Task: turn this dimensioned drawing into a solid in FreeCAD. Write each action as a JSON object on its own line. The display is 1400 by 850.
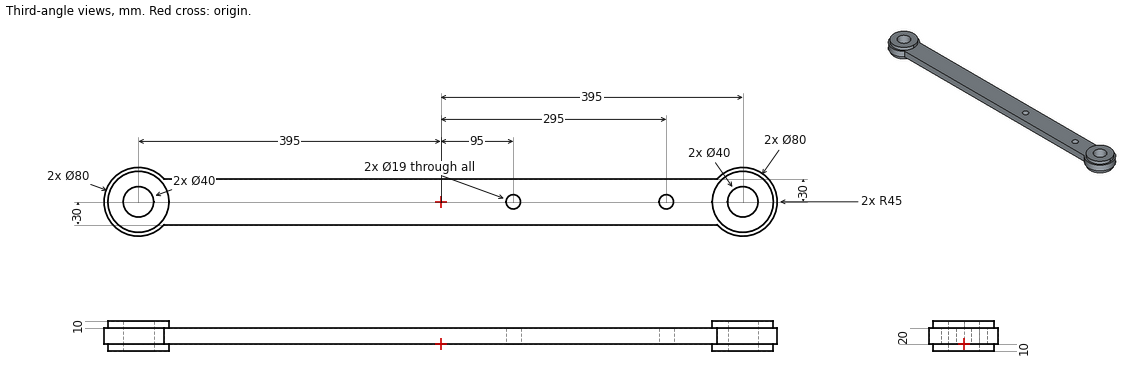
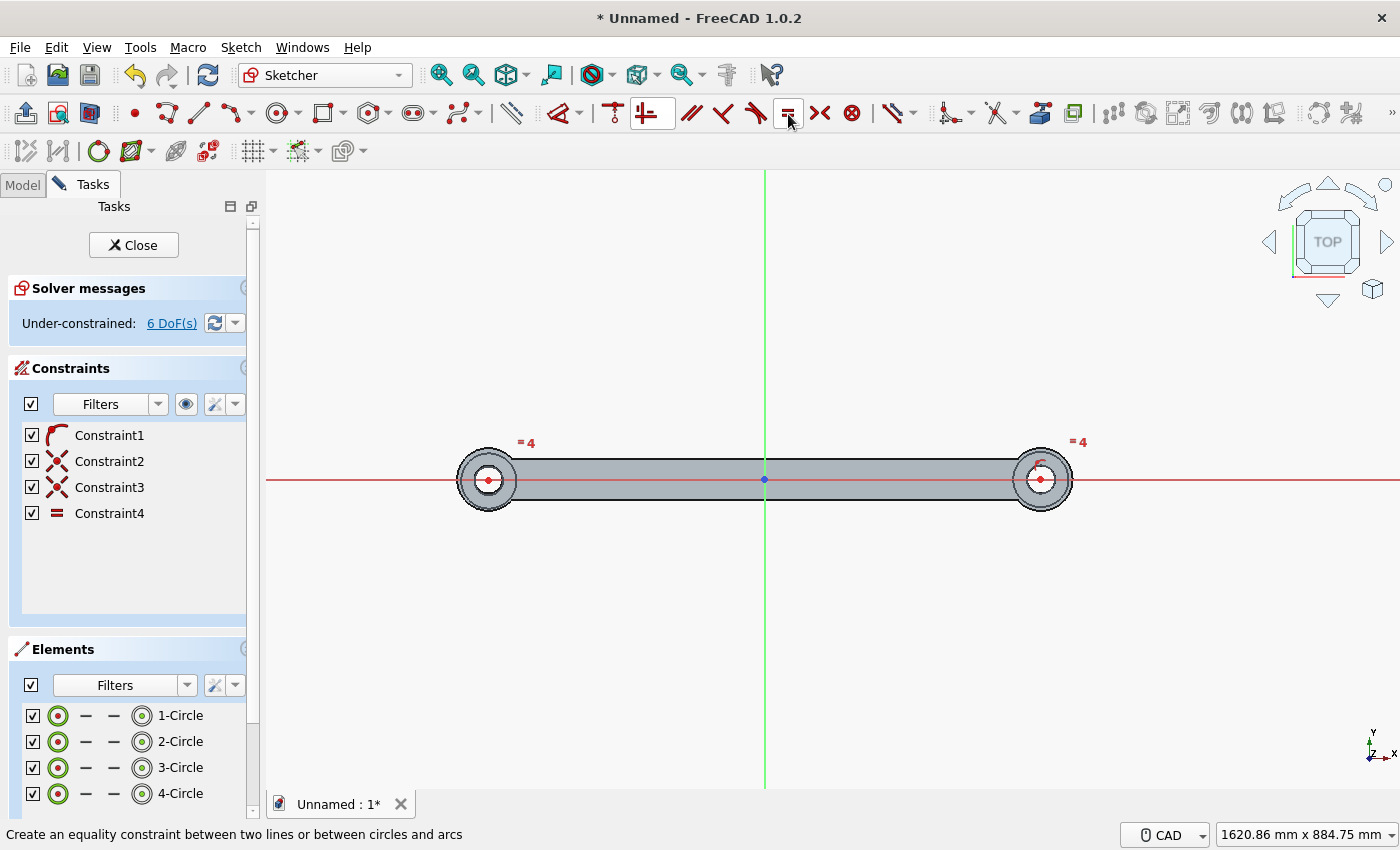
{"action": "left_click", "coordinate": [479, 491]}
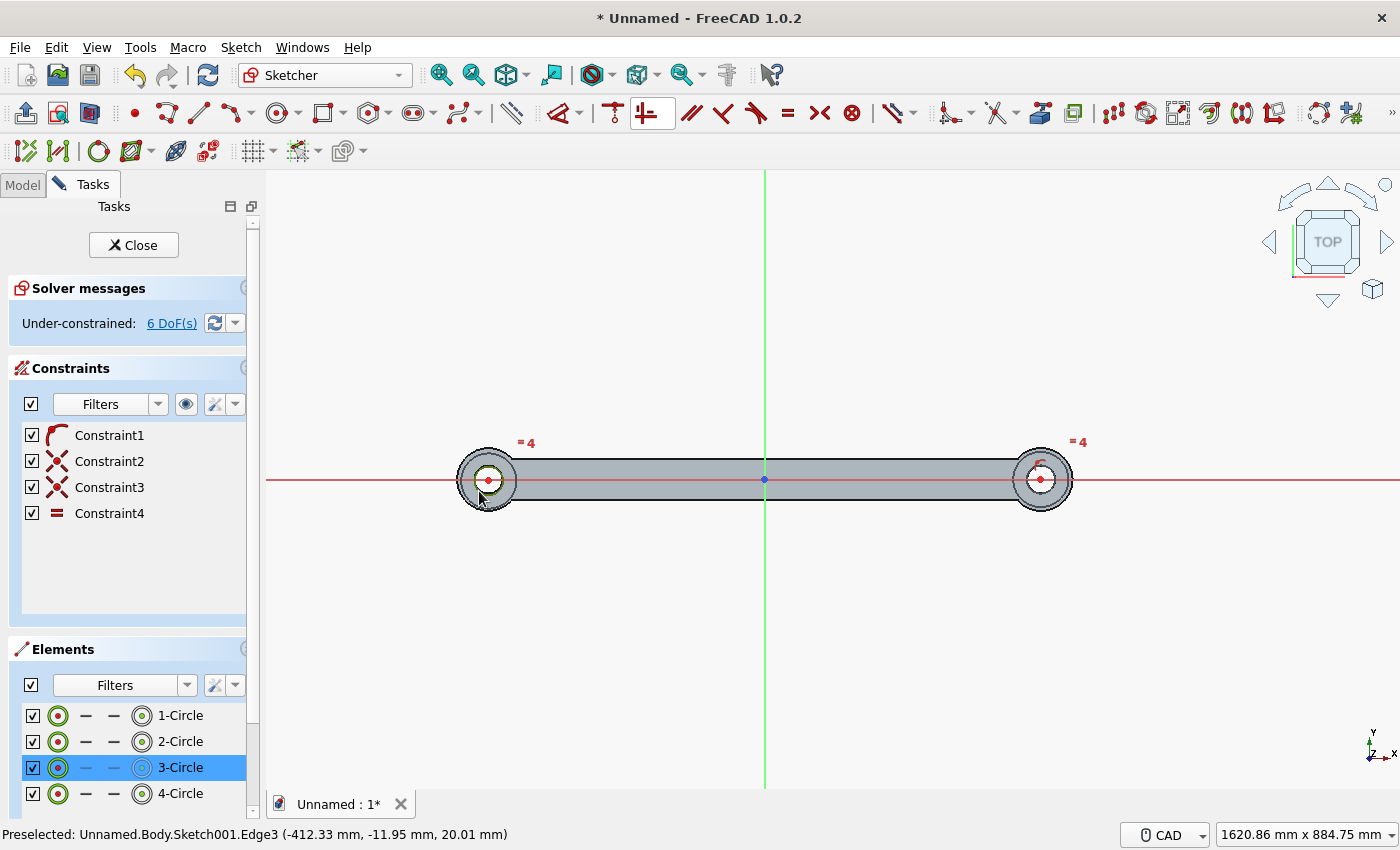
{"action": "scroll", "coordinate": [1051, 470], "scroll_direction": "up", "scroll_amount": 2}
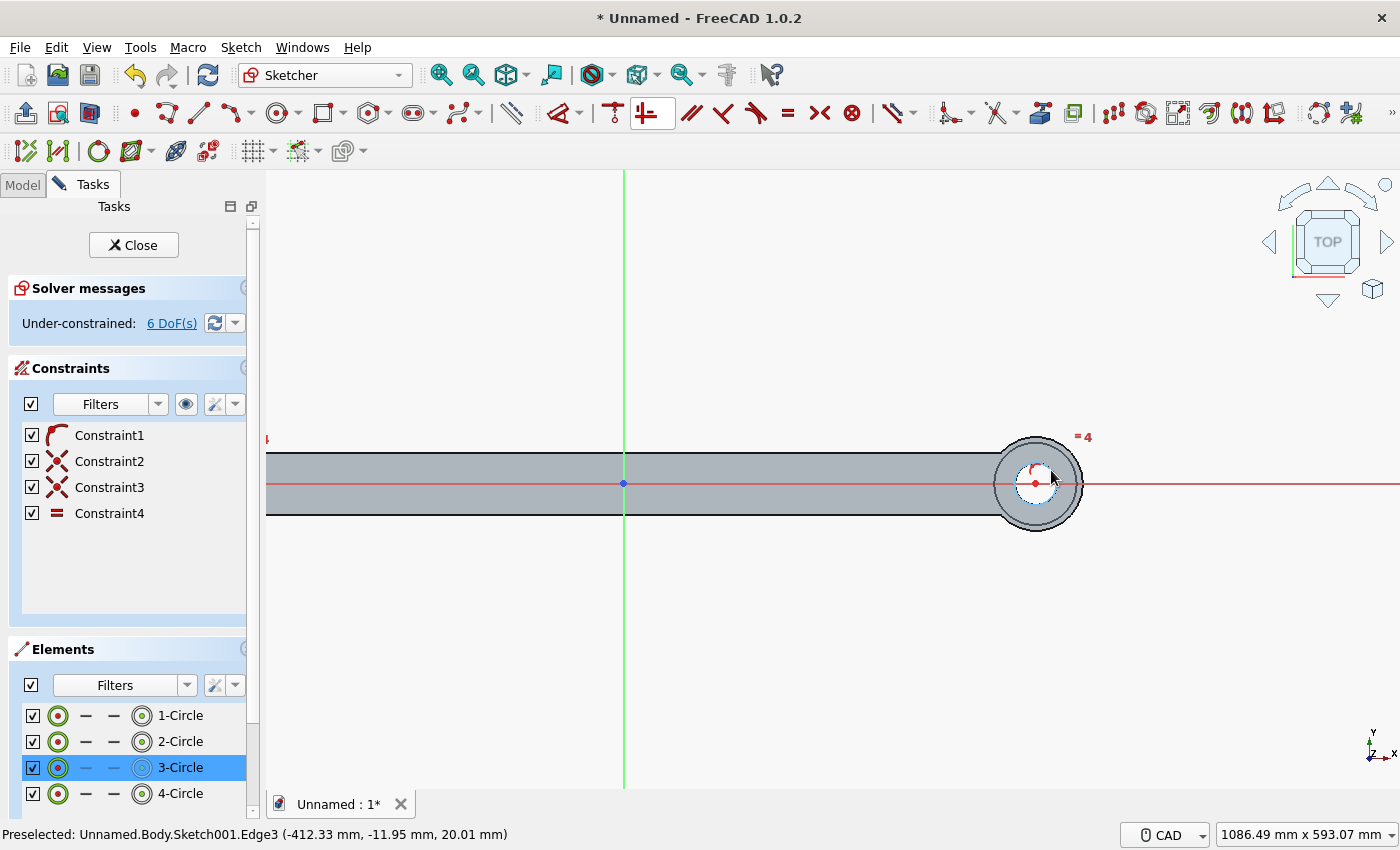
{"action": "left_click", "coordinate": [1050, 469]}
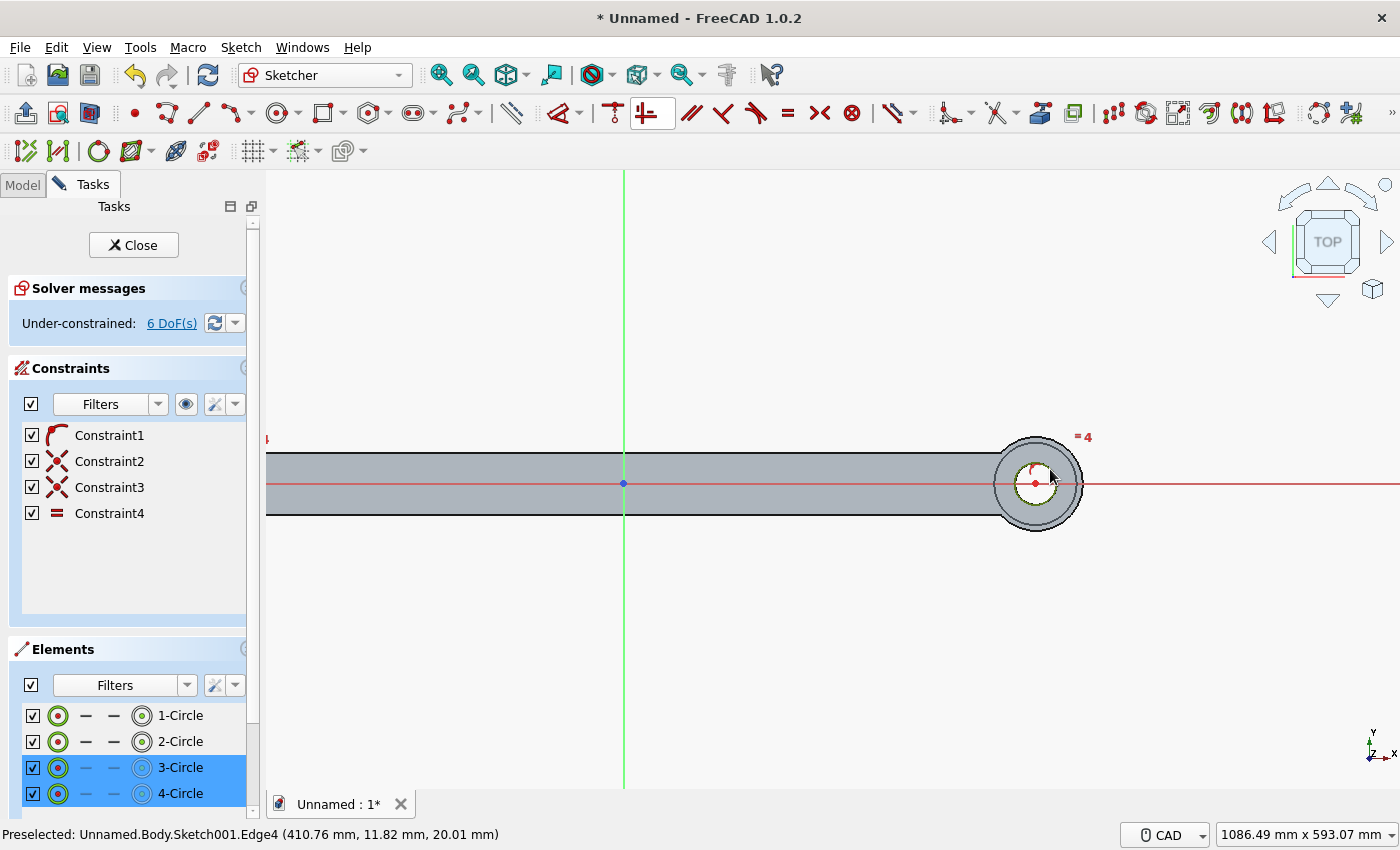
{"action": "left_click", "coordinate": [788, 114]}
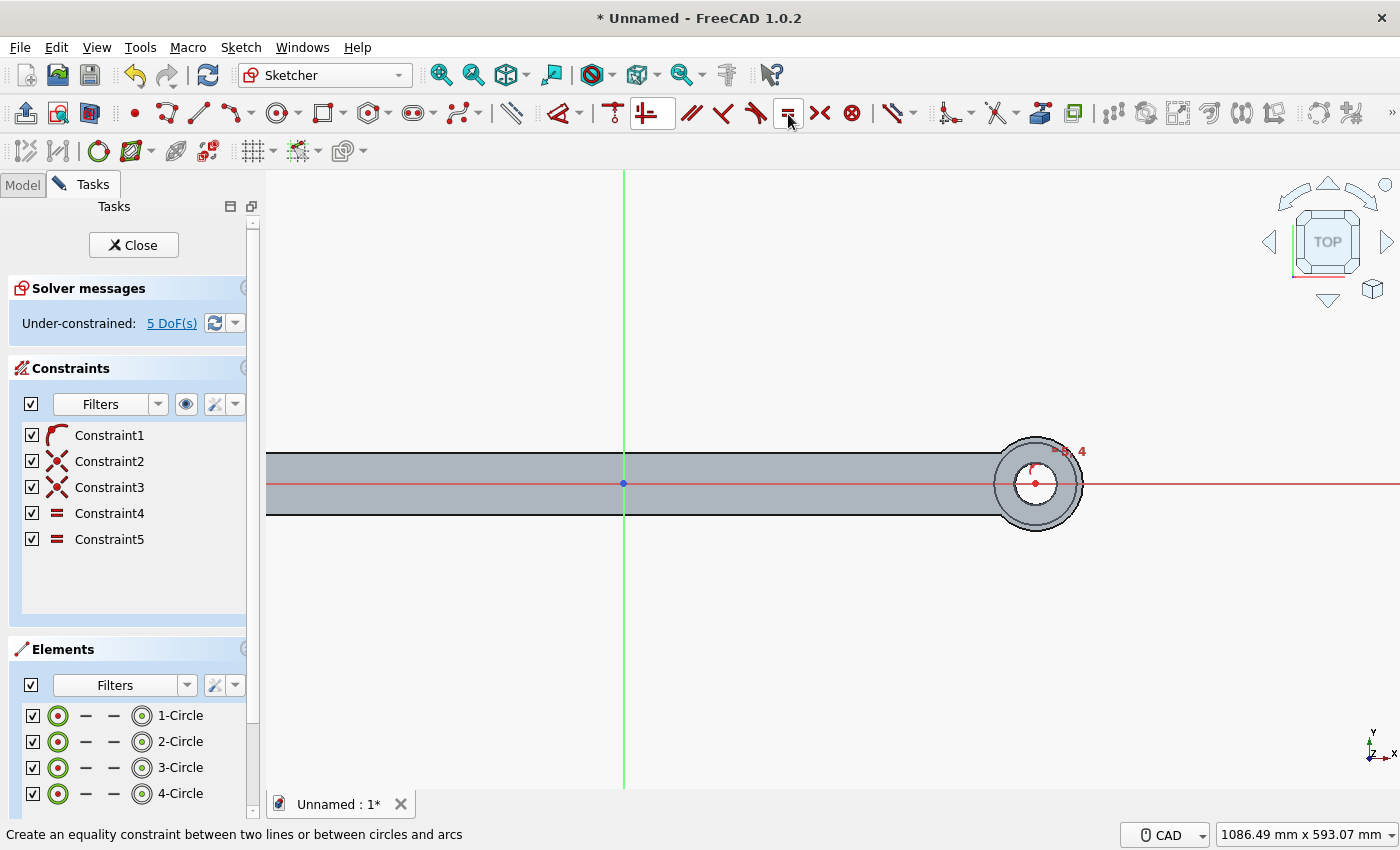
{"action": "scroll", "coordinate": [1051, 470], "scroll_direction": "down", "scroll_amount": 2}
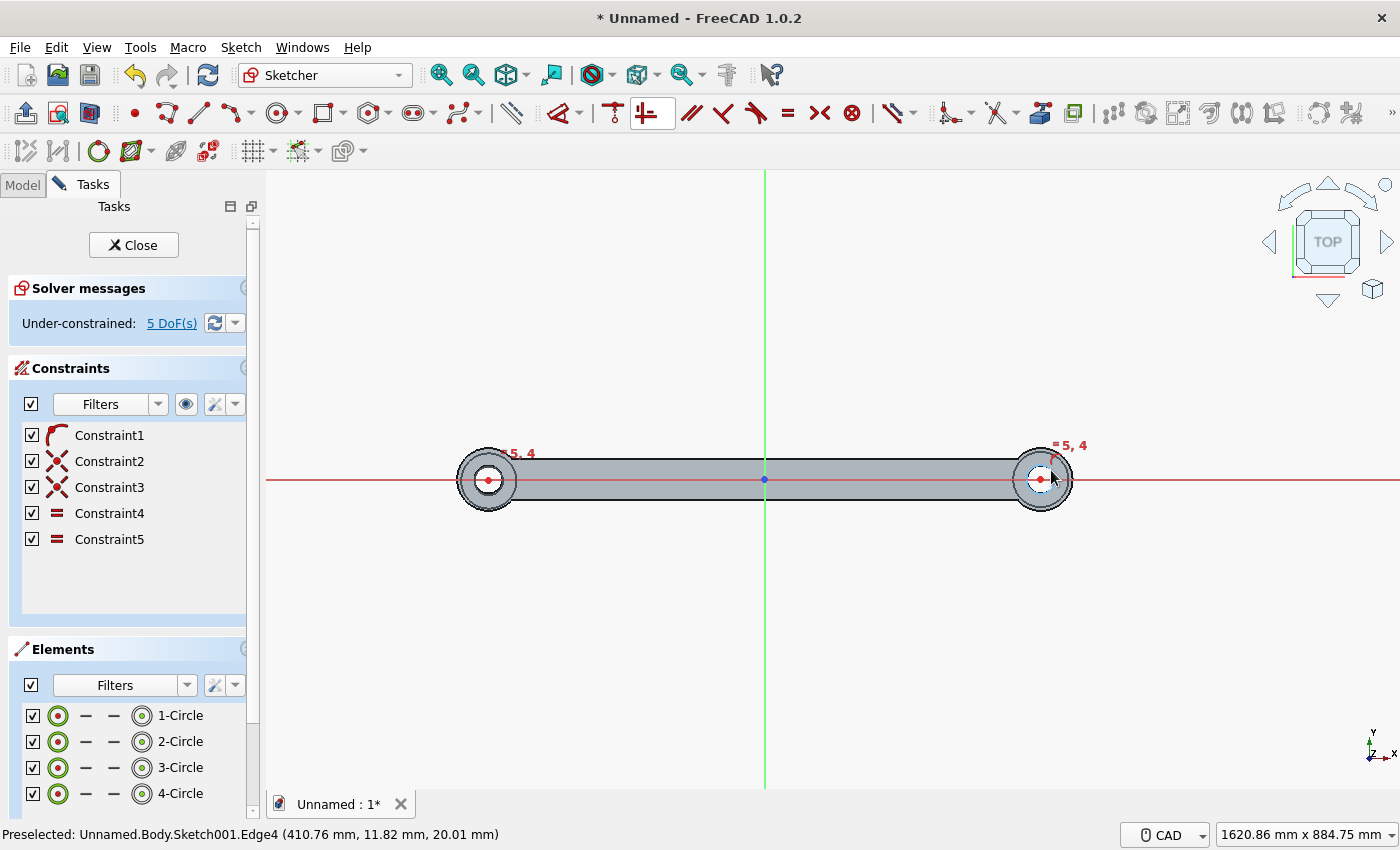
{"action": "left_click", "coordinate": [489, 481]}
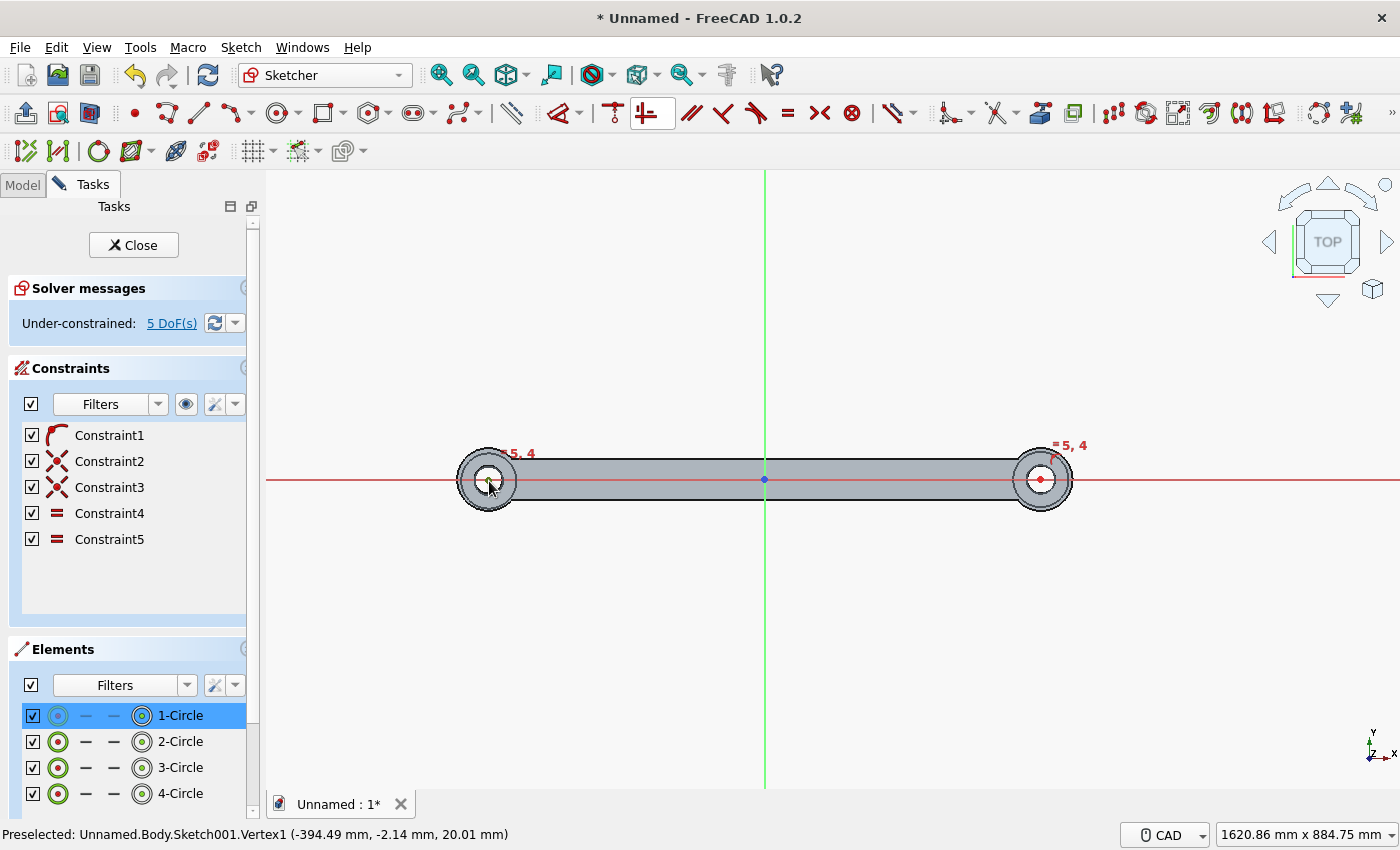
{"action": "left_click", "coordinate": [361, 480]}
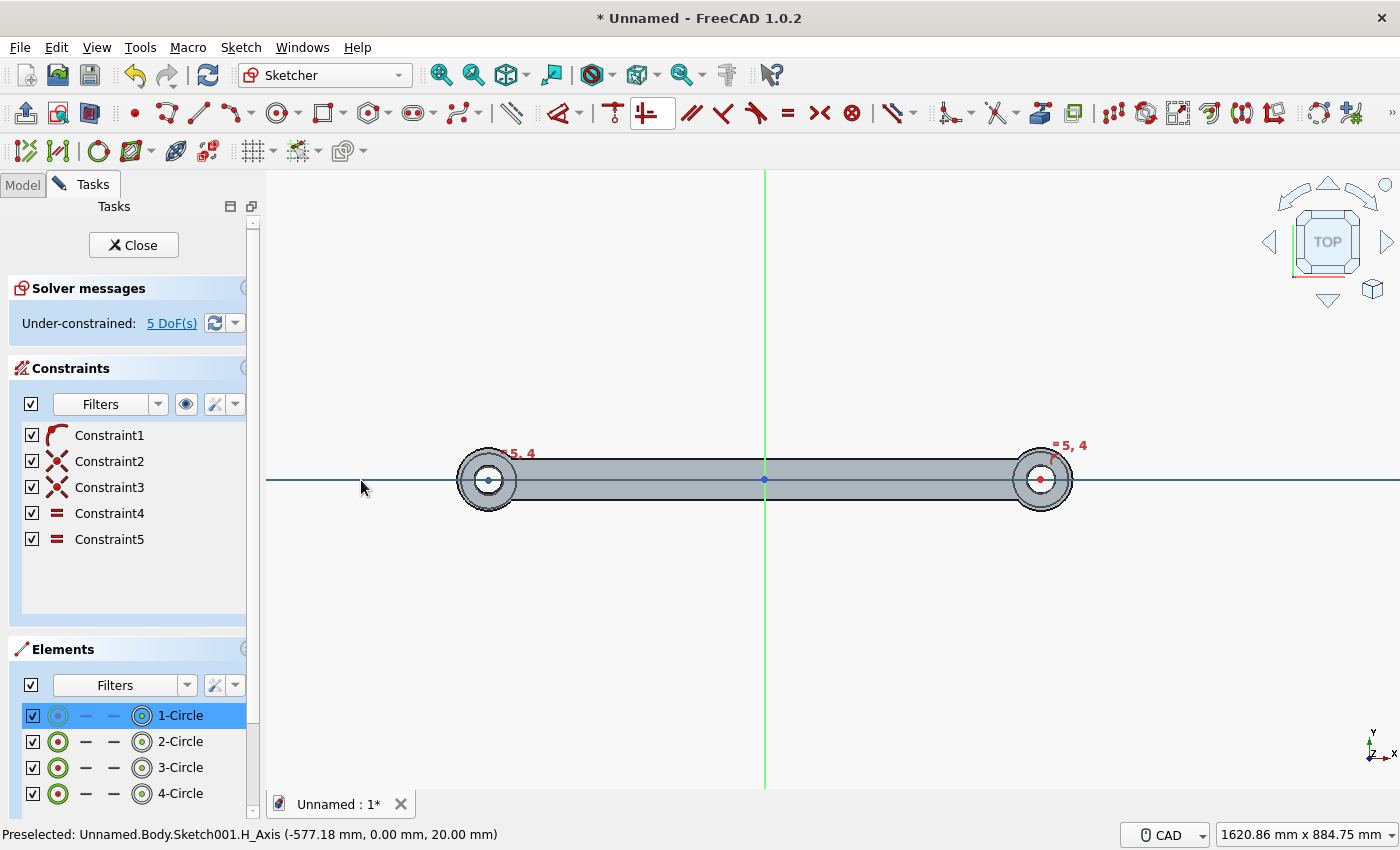
{"action": "left_click", "coordinate": [614, 114]}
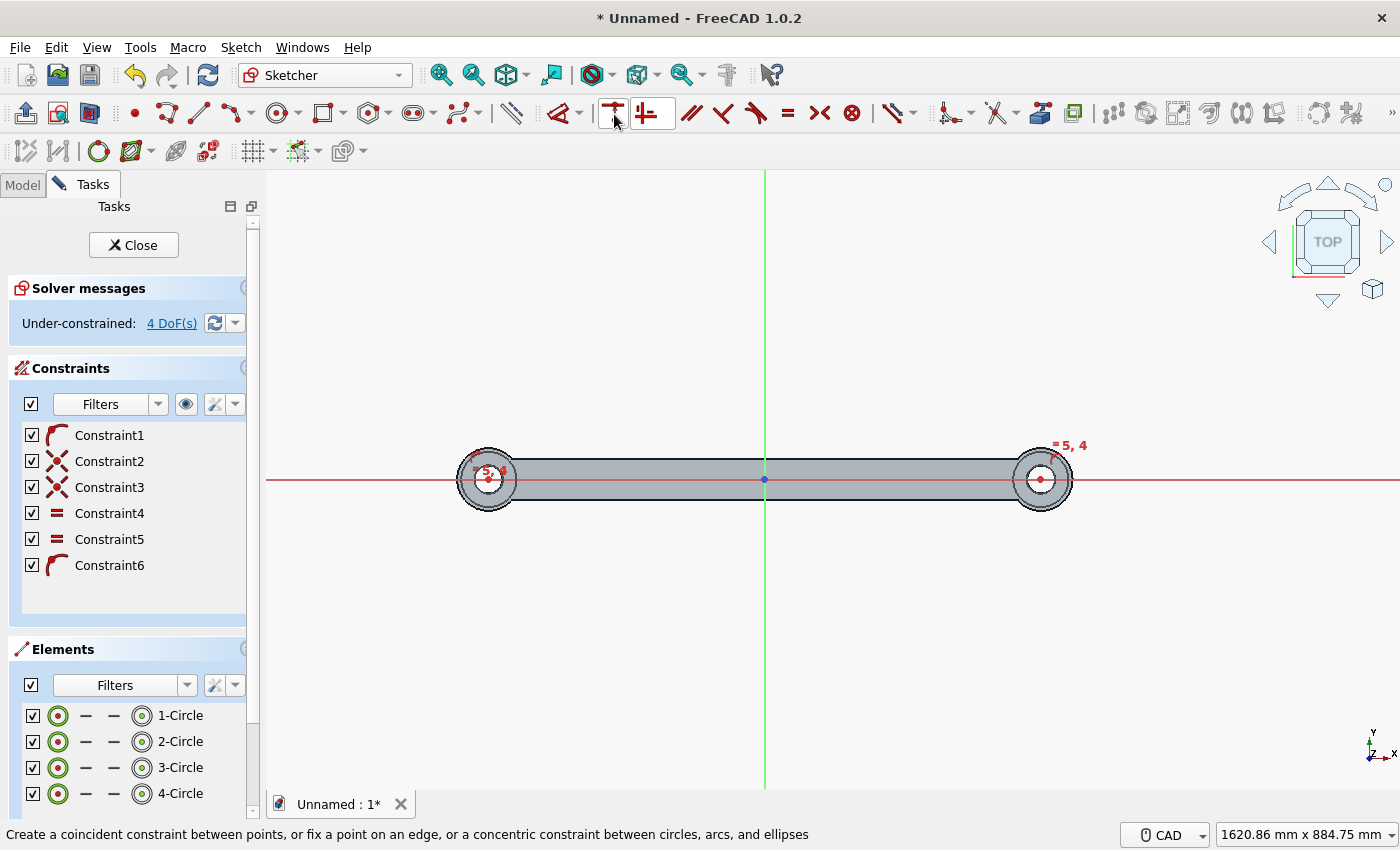
{"action": "left_click", "coordinate": [558, 114]}